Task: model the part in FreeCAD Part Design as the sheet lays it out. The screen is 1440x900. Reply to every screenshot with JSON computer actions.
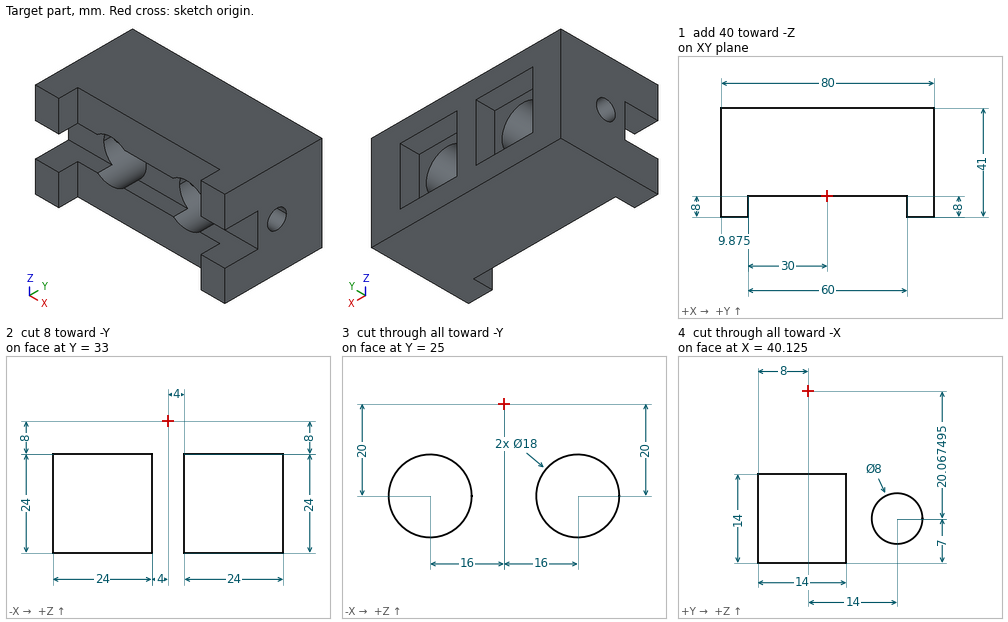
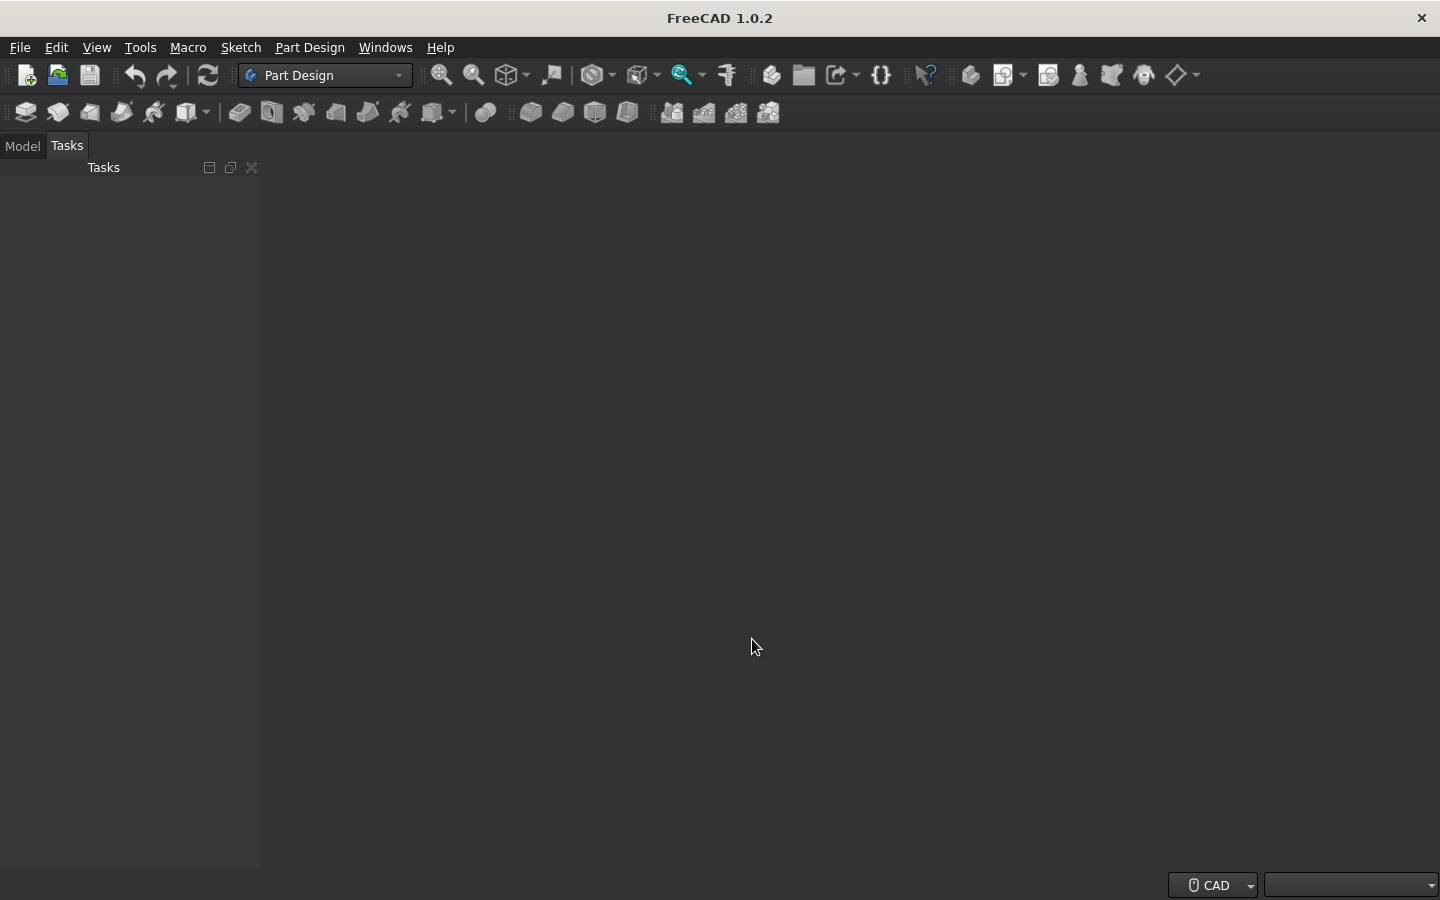
{"action": "left_click", "coordinate": [26, 76]}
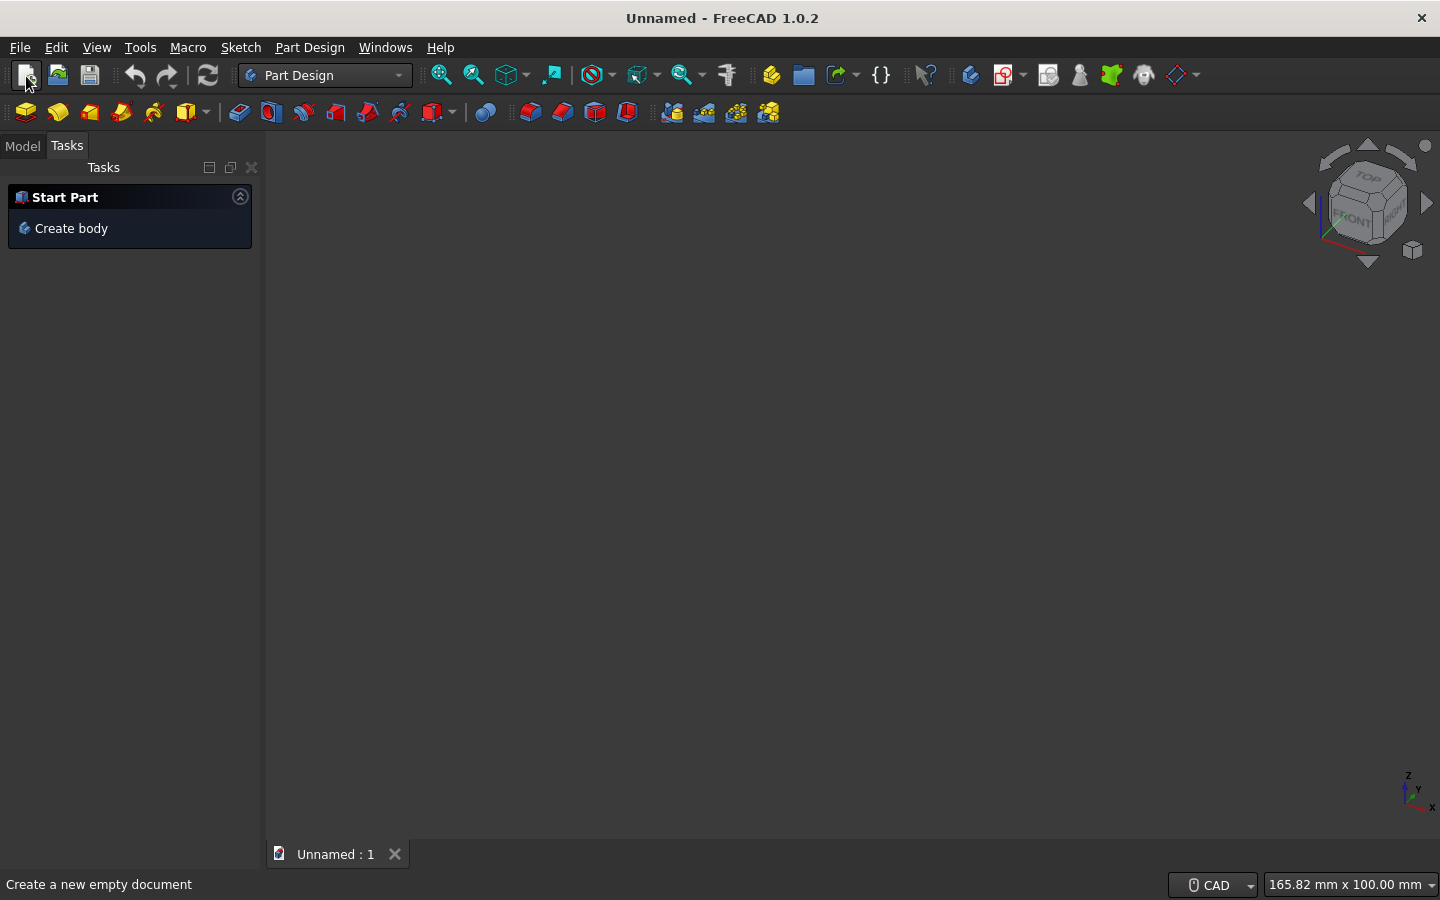
{"action": "left_click", "coordinate": [1004, 76]}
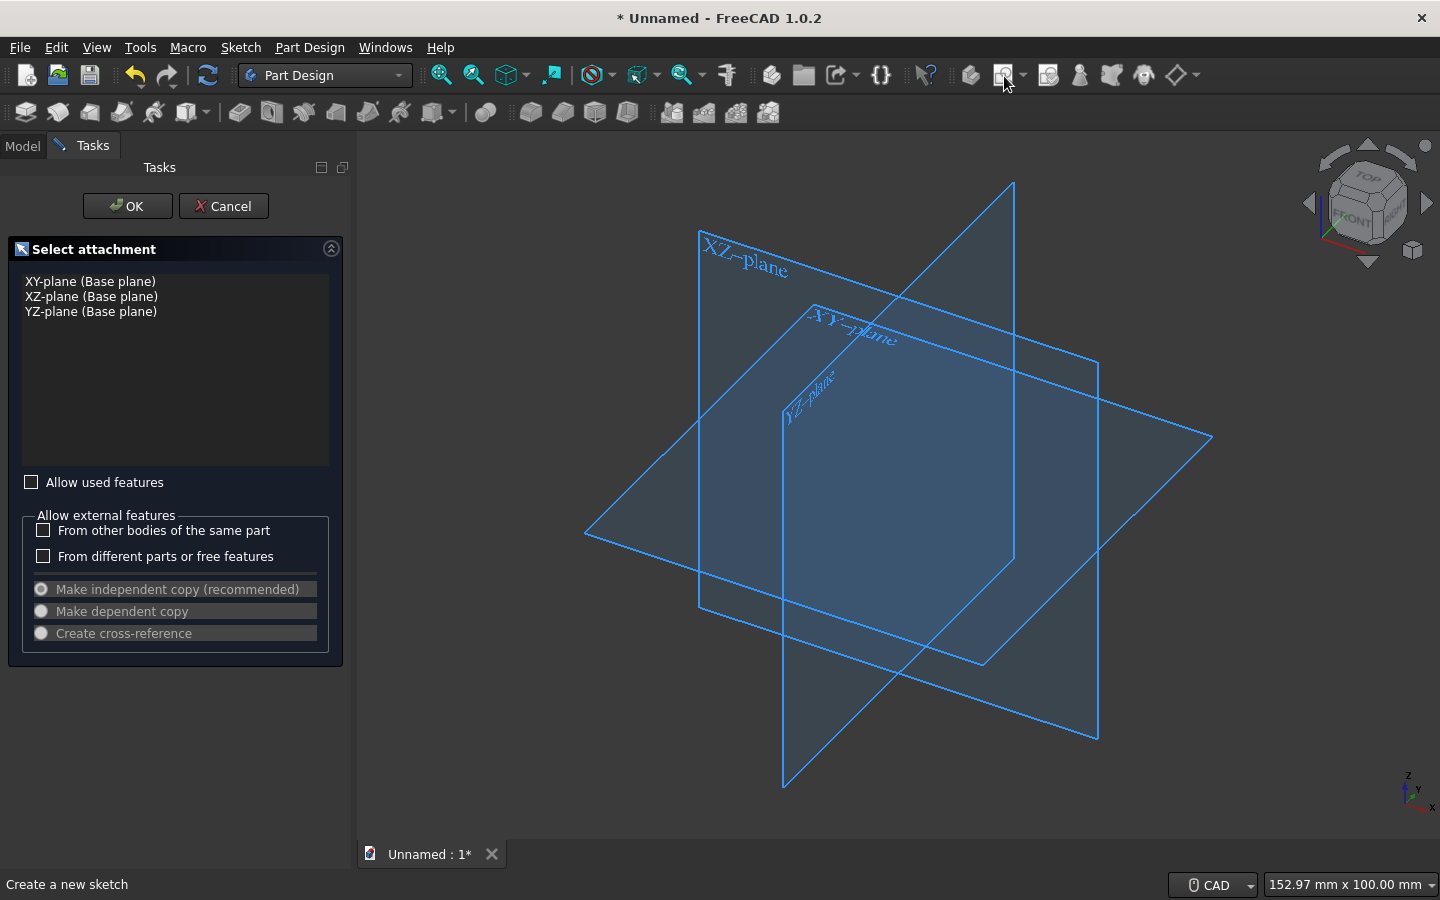
{"action": "left_click", "coordinate": [82, 282]}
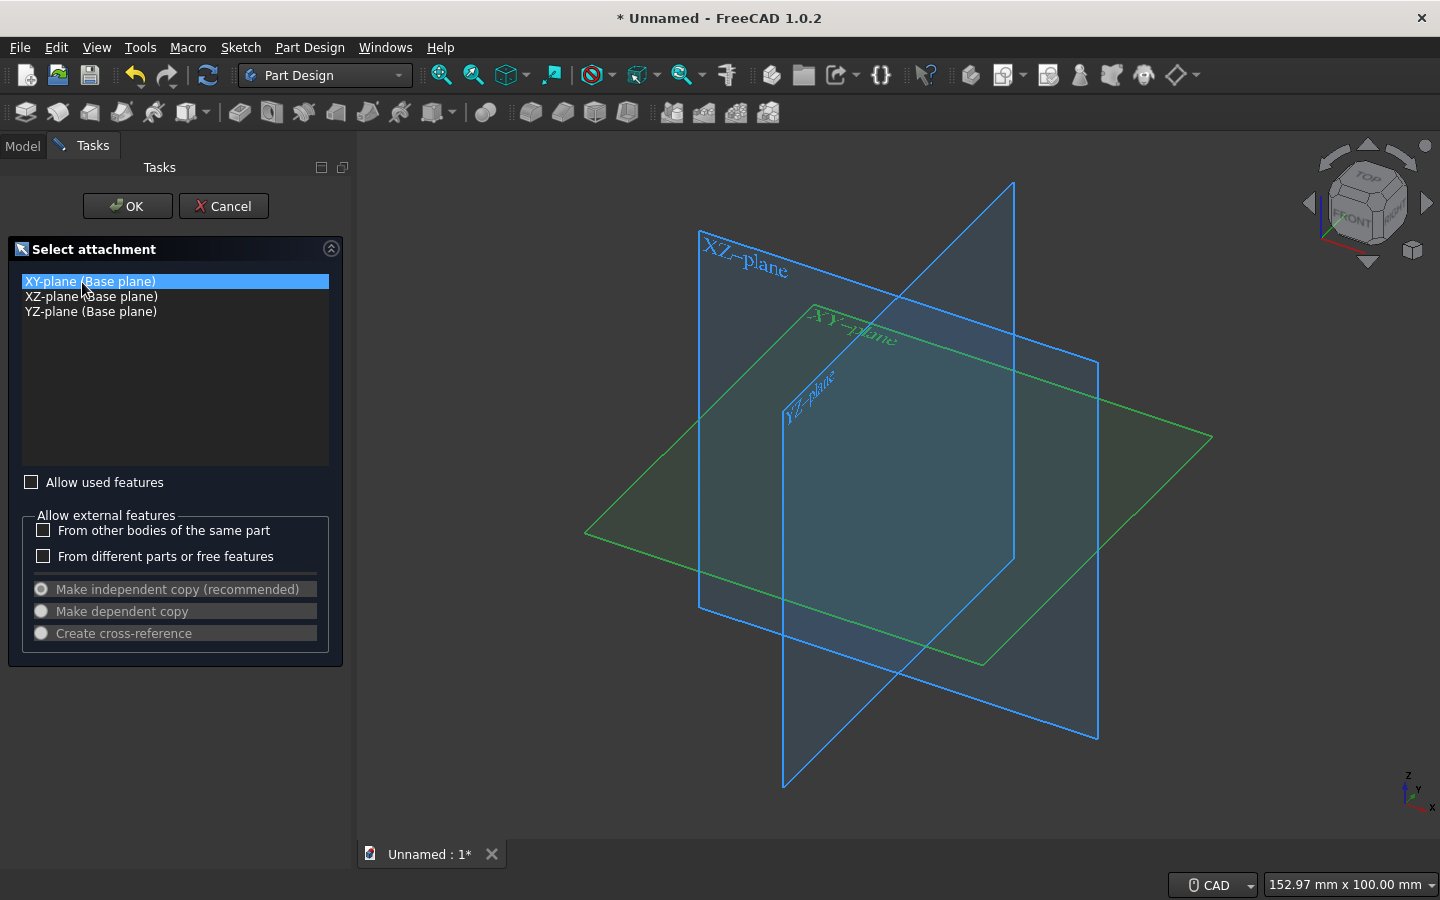
{"action": "left_click", "coordinate": [128, 206]}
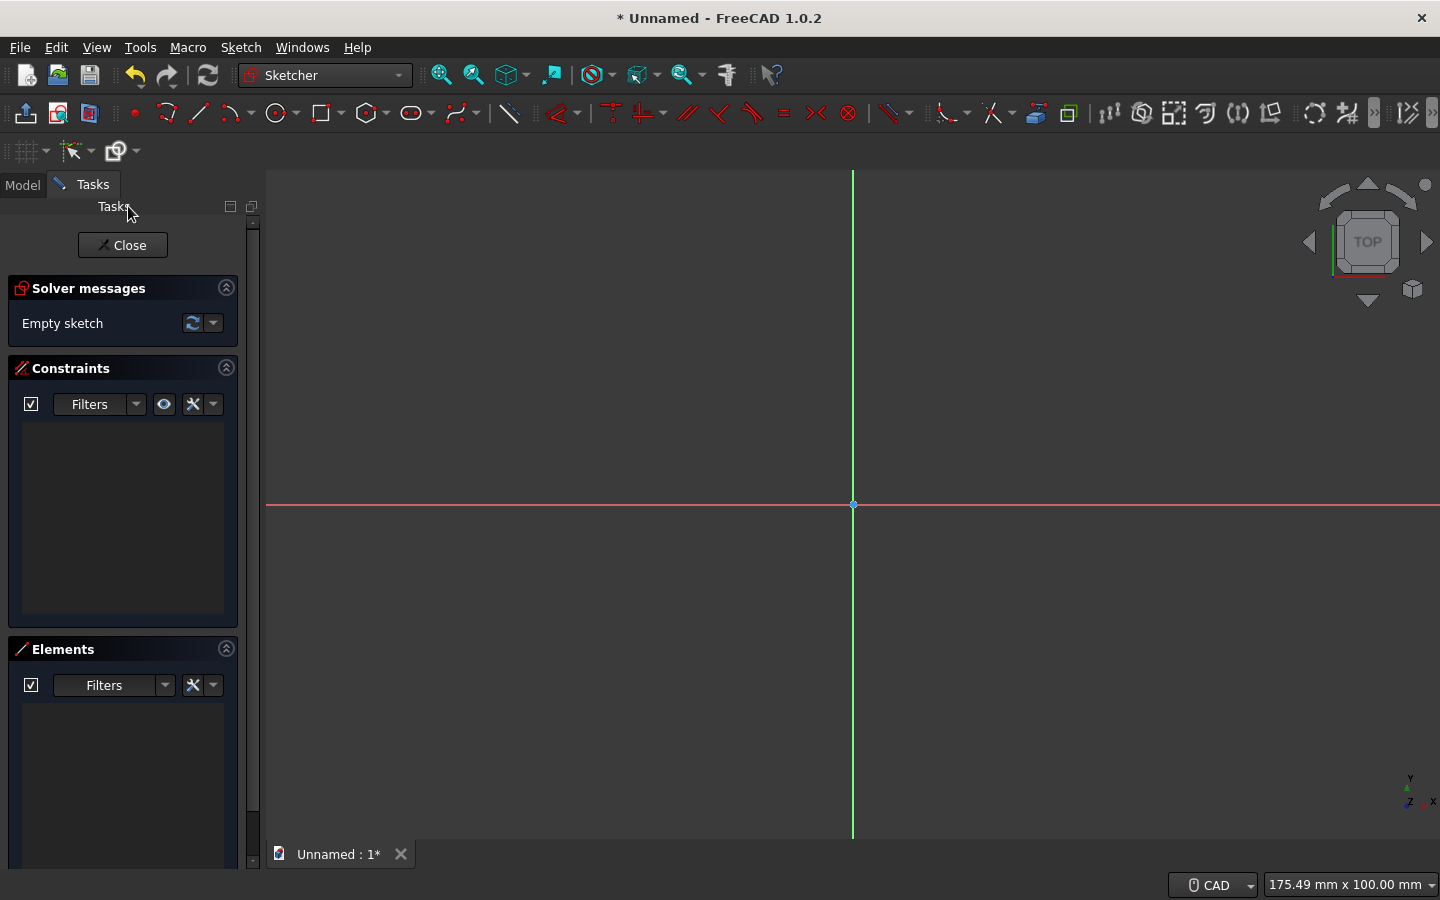
{"action": "left_click", "coordinate": [168, 114]}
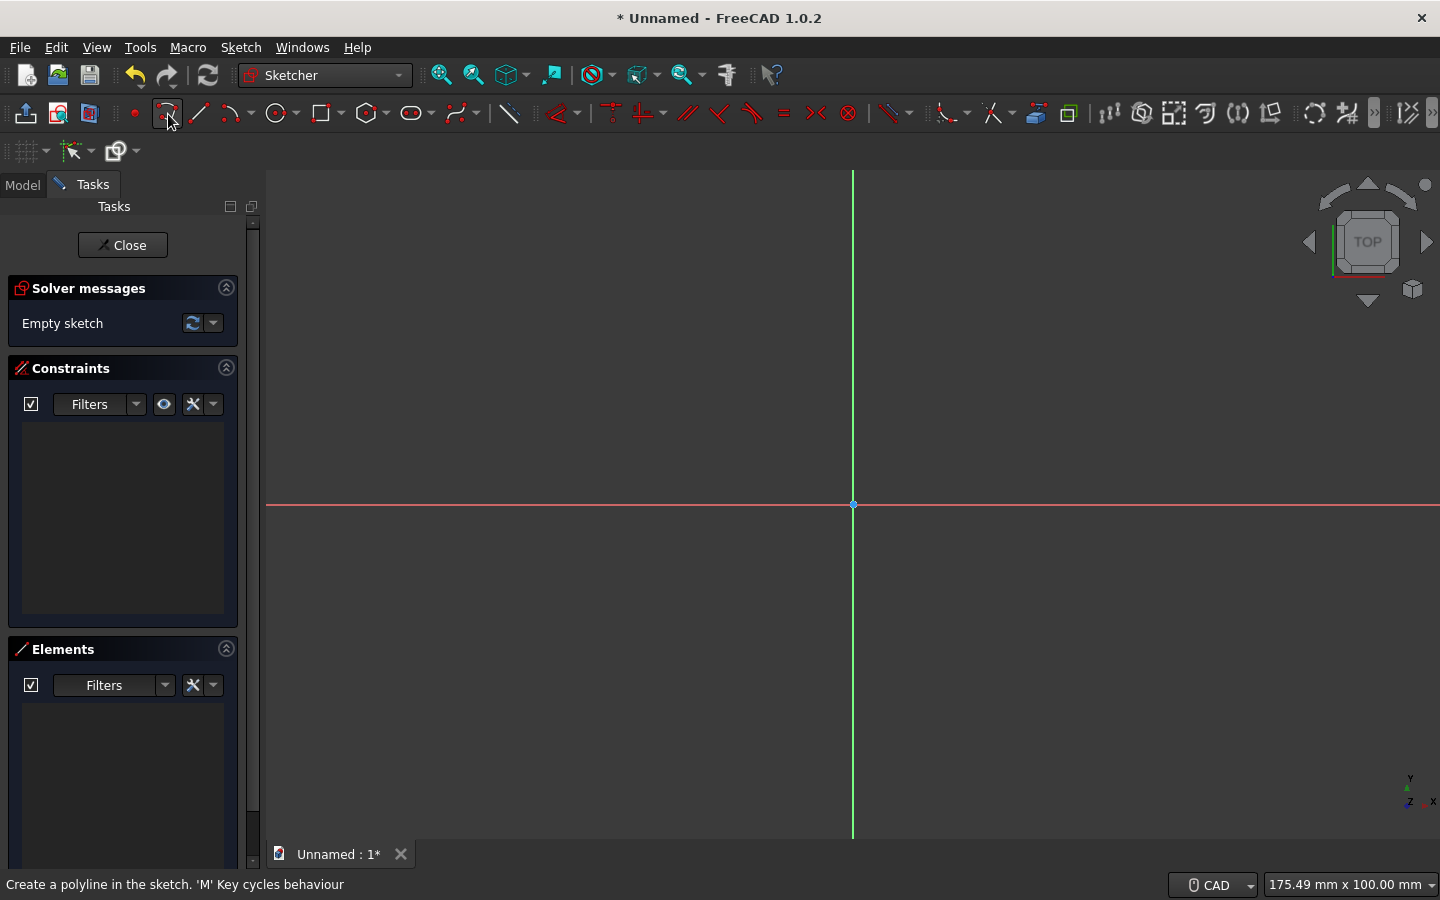
{"action": "left_click", "coordinate": [652, 504]}
{"action": "left_click", "coordinate": [1054, 496]}
{"action": "left_click", "coordinate": [1054, 558]}
{"action": "left_click", "coordinate": [1121, 558]}
{"action": "left_click", "coordinate": [1121, 284]}
{"action": "left_click", "coordinate": [586, 284]}
{"action": "left_click", "coordinate": [586, 558]}
{"action": "left_click", "coordinate": [652, 558]}
{"action": "left_click", "coordinate": [652, 504]}
{"action": "key", "text": "Escape"}
{"action": "key", "text": "Escape"}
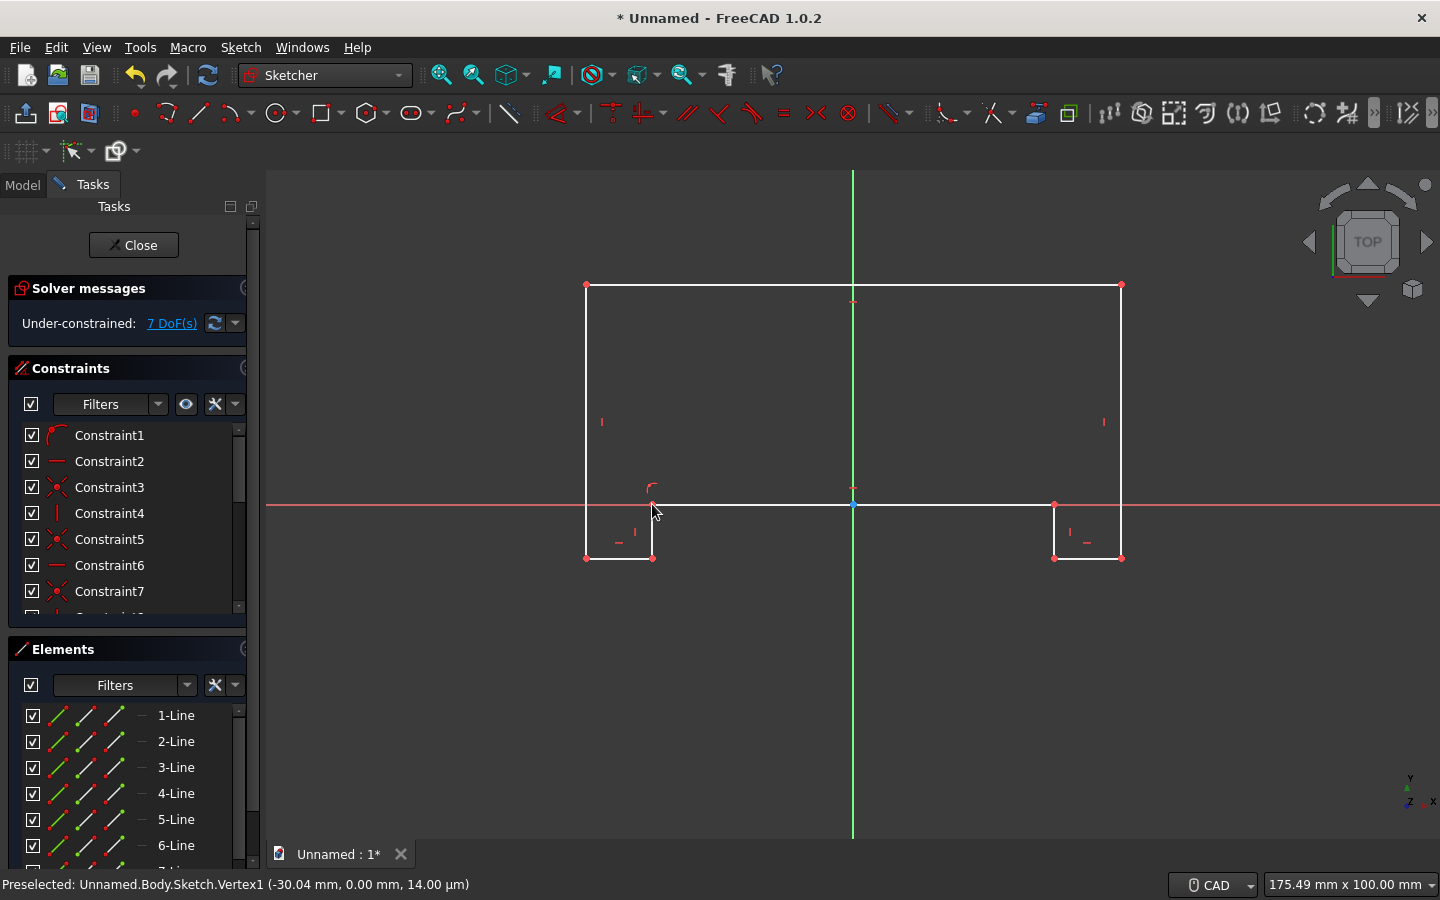
{"action": "left_click", "coordinate": [556, 114]}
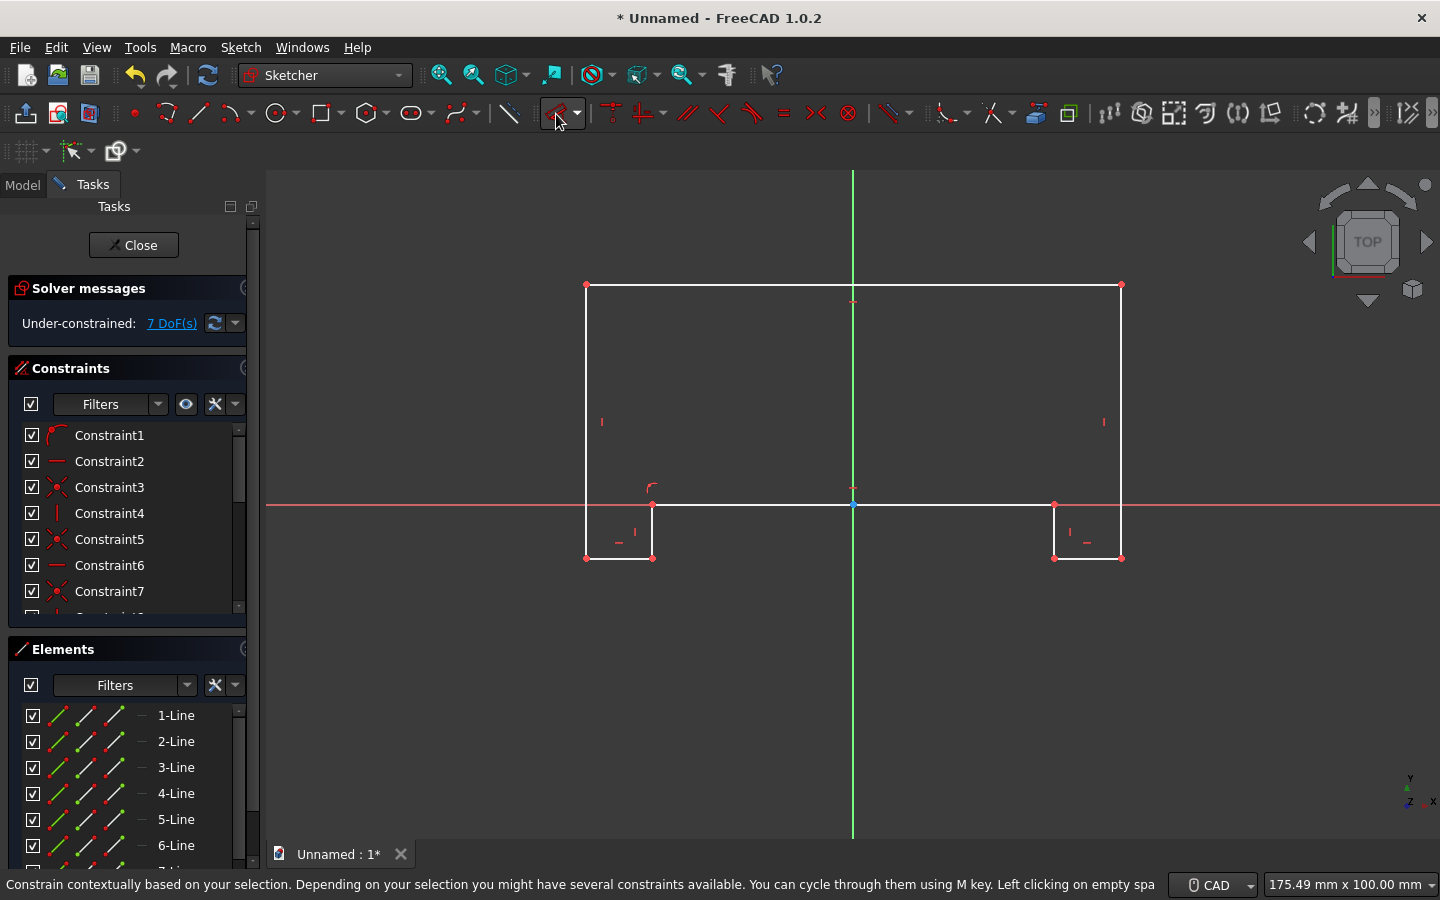
{"action": "left_click", "coordinate": [1054, 521]}
{"action": "left_click", "coordinate": [1088, 532]}